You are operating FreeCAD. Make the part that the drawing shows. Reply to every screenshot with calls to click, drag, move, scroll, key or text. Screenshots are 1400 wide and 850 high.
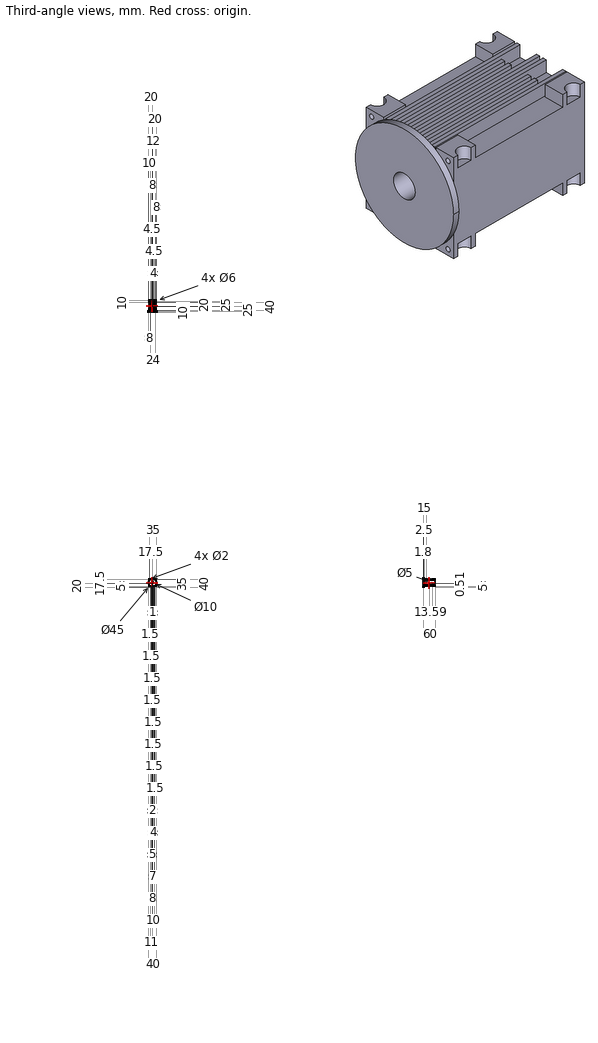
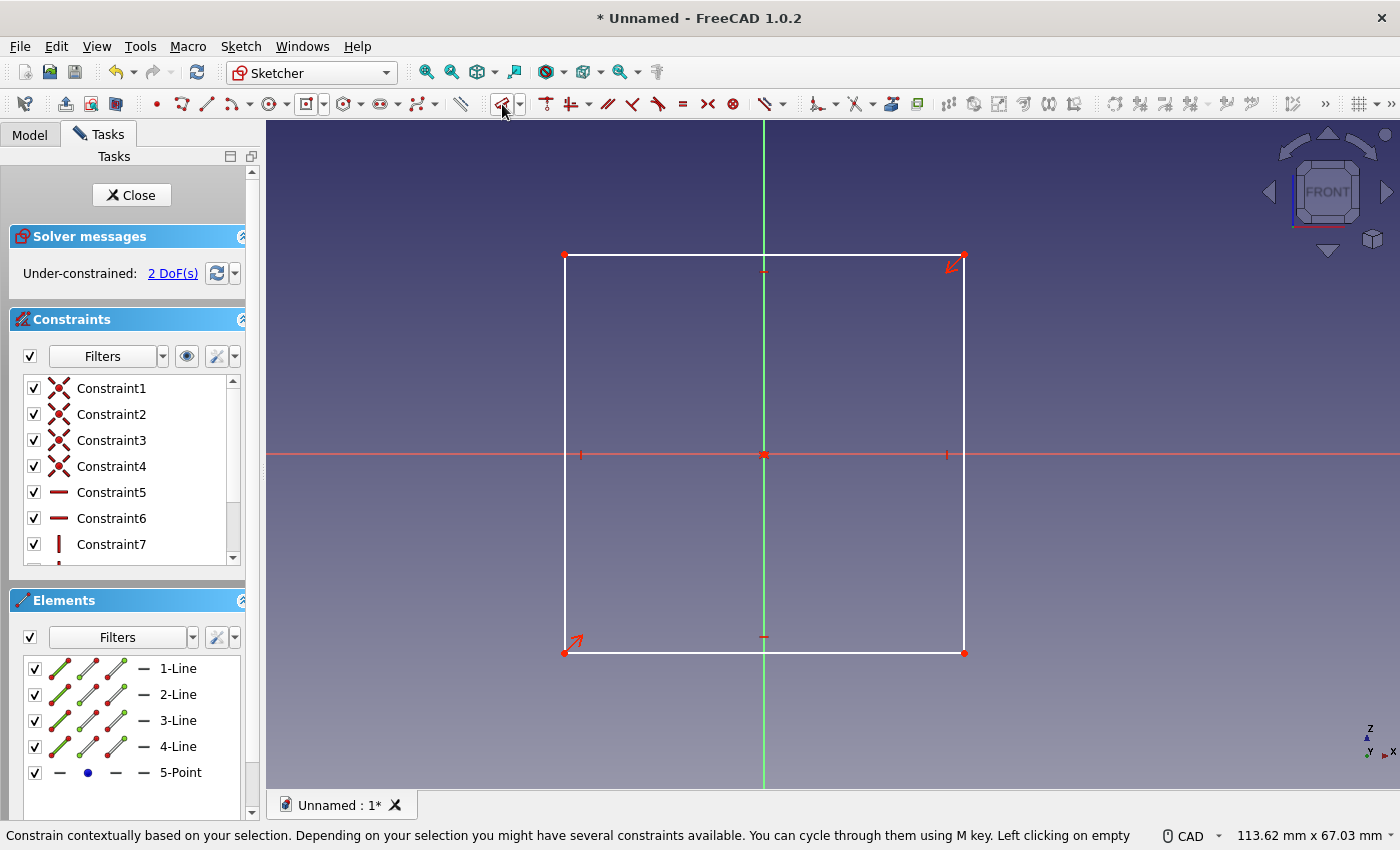
click(684, 653)
click(672, 687)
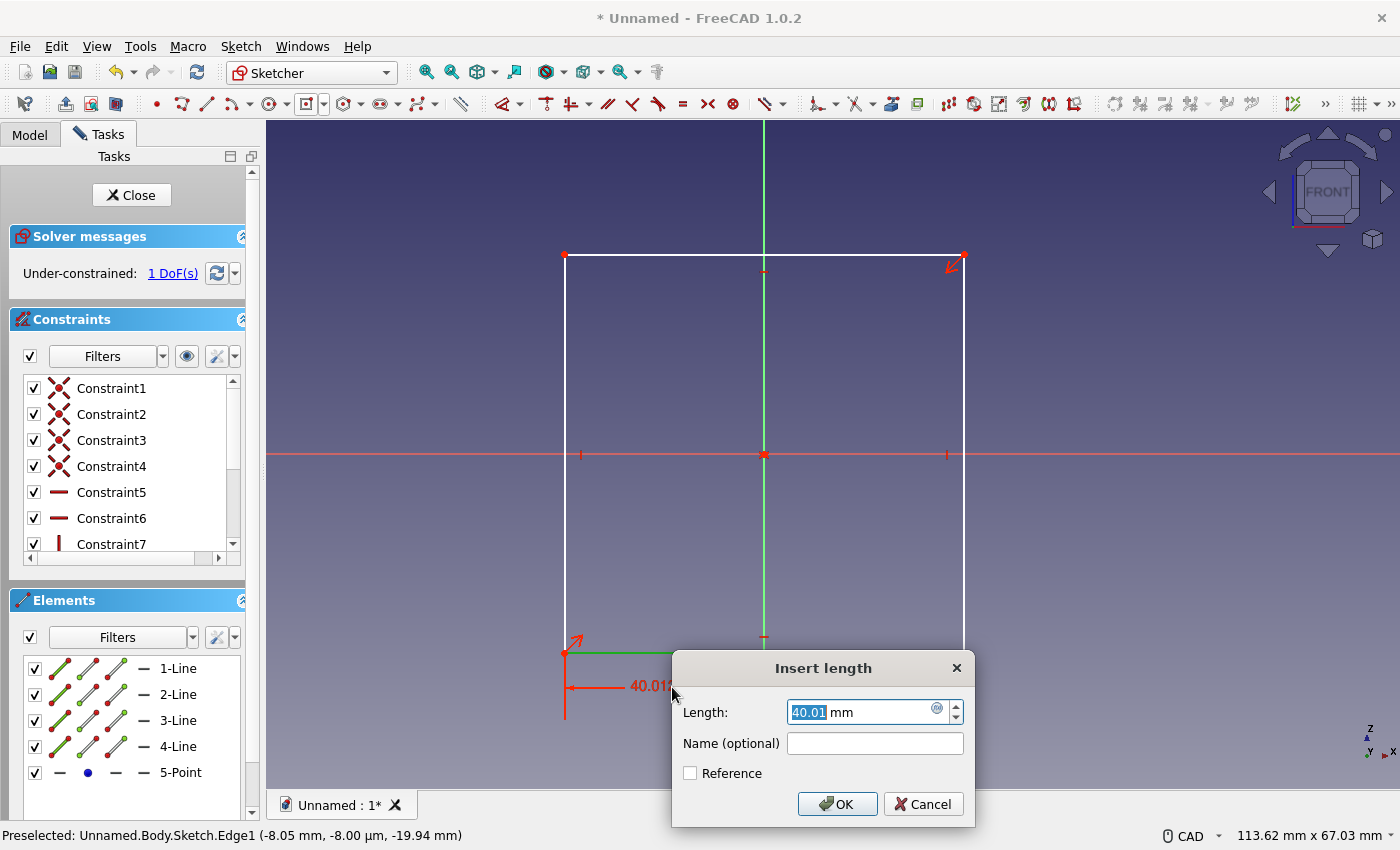
text(40)
key(Return)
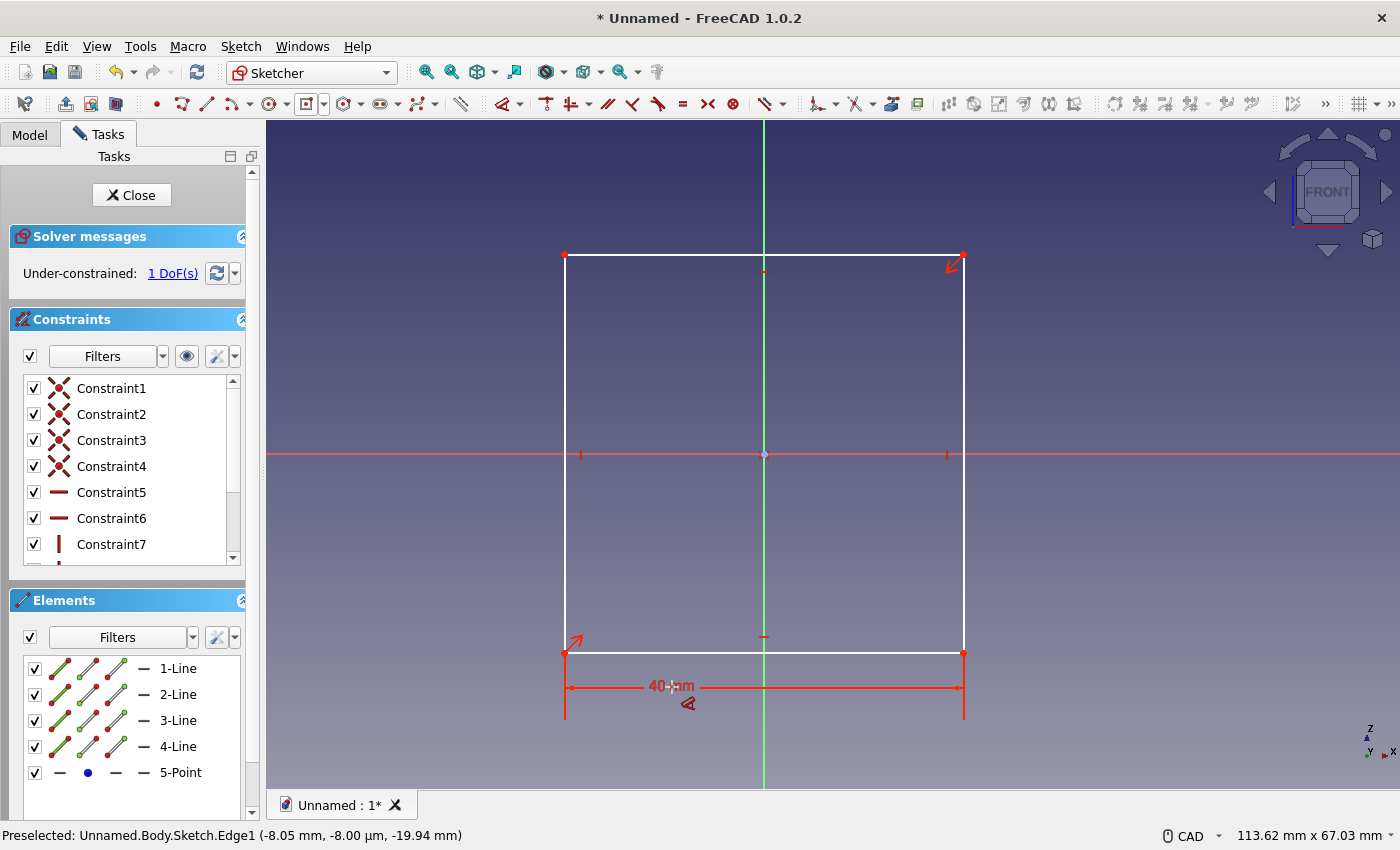
click(964, 534)
click(998, 362)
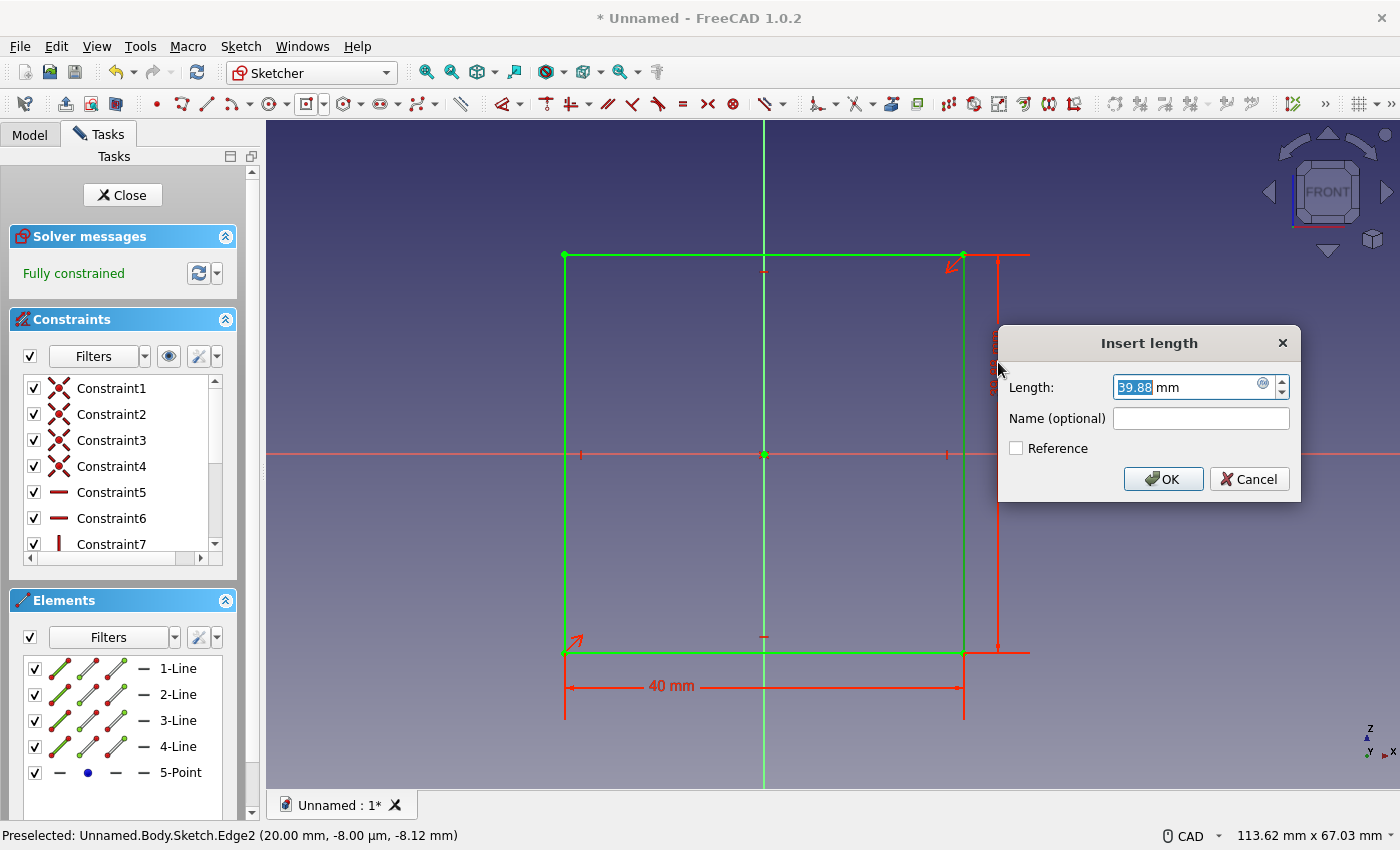
text(40)
key(Return)
key(Escape)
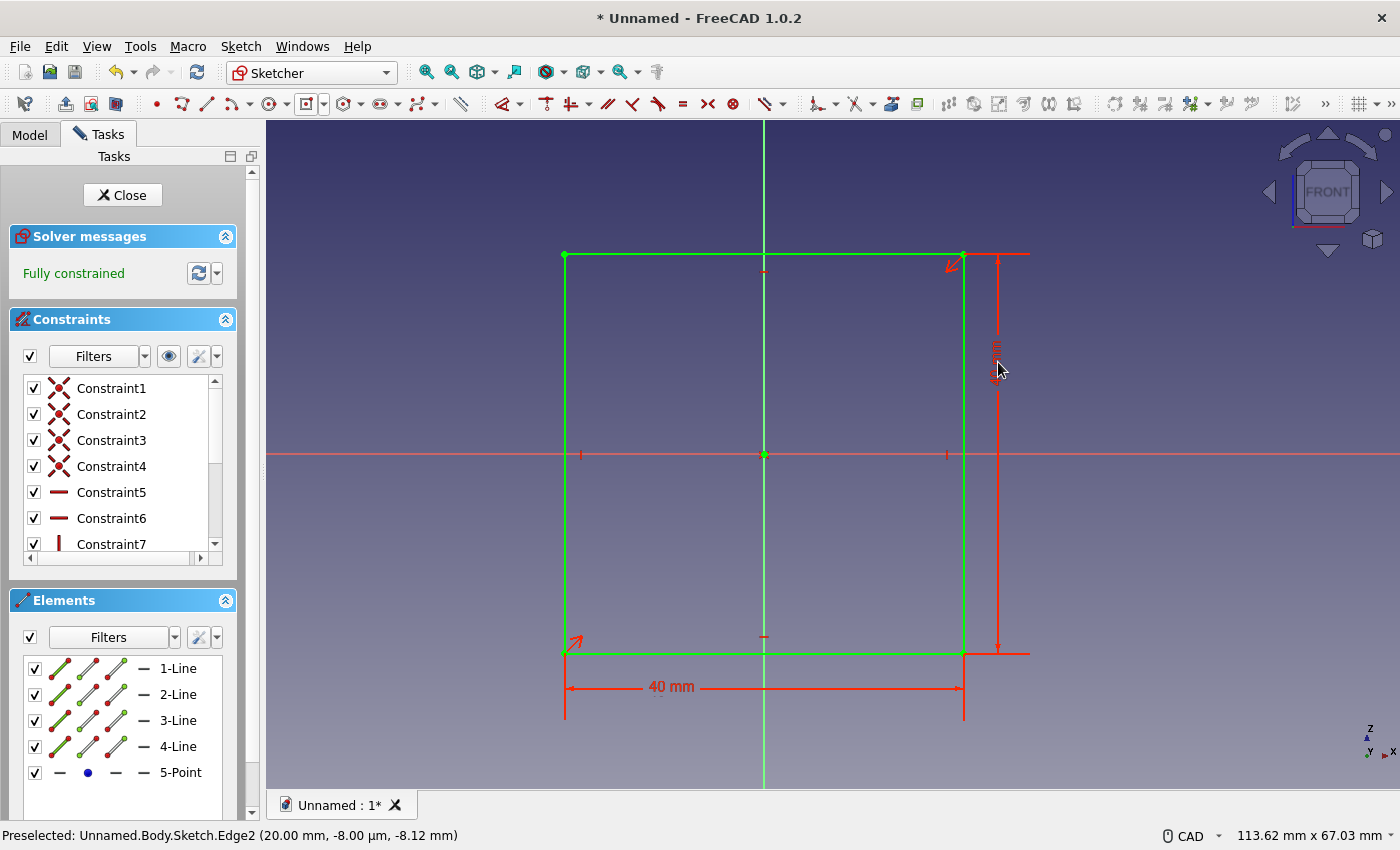
click(123, 195)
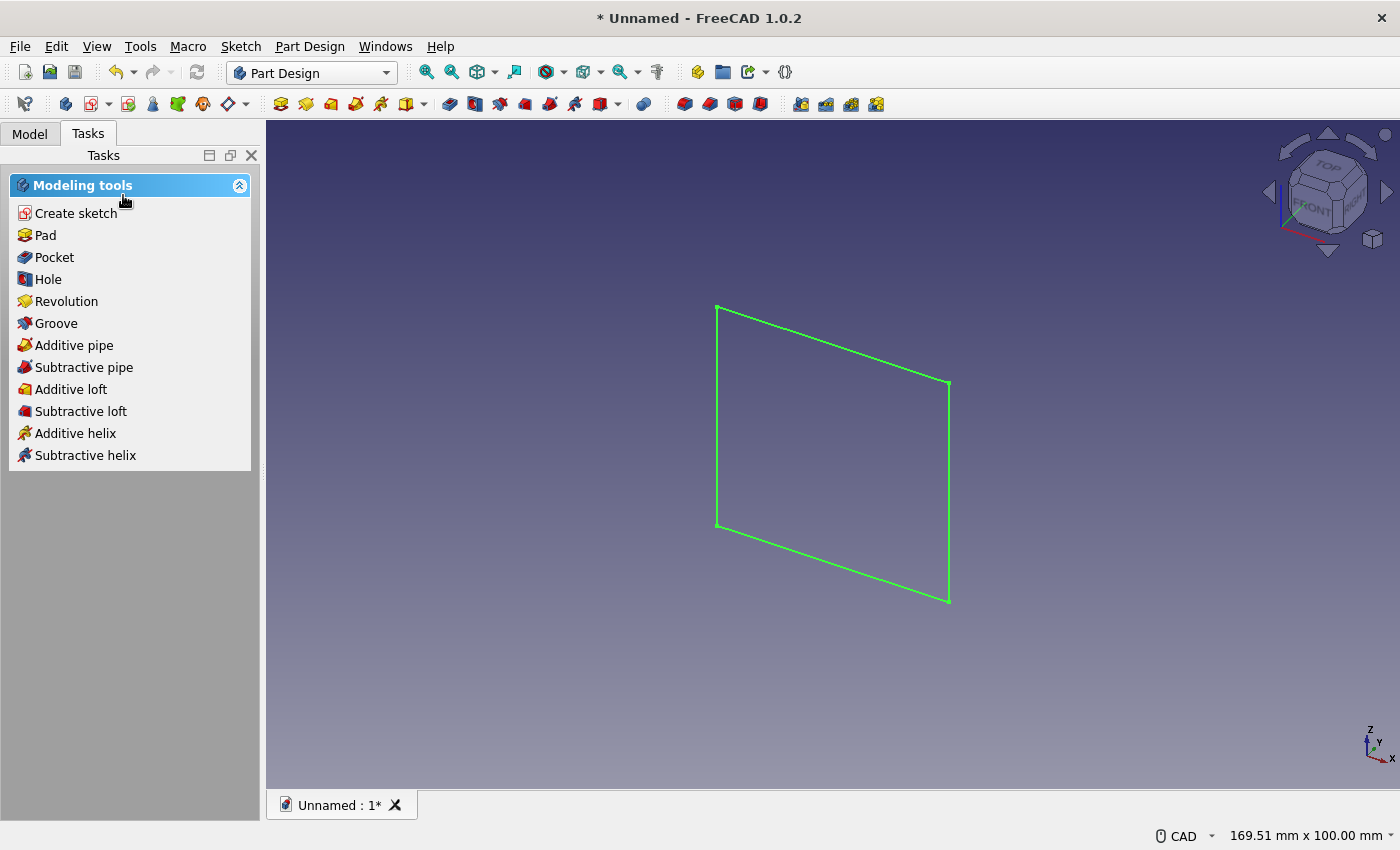
click(281, 104)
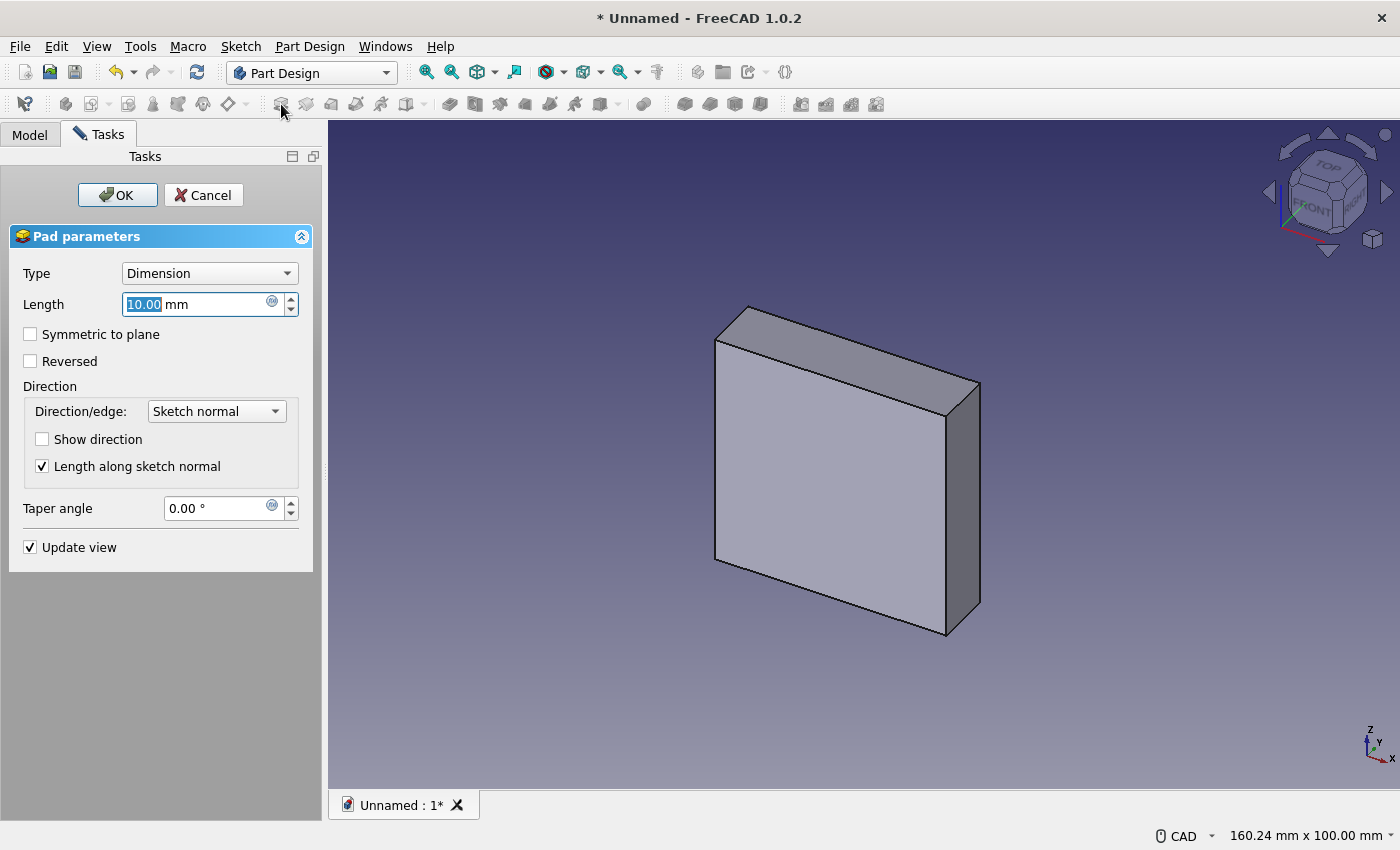
text(60)
key(Tab)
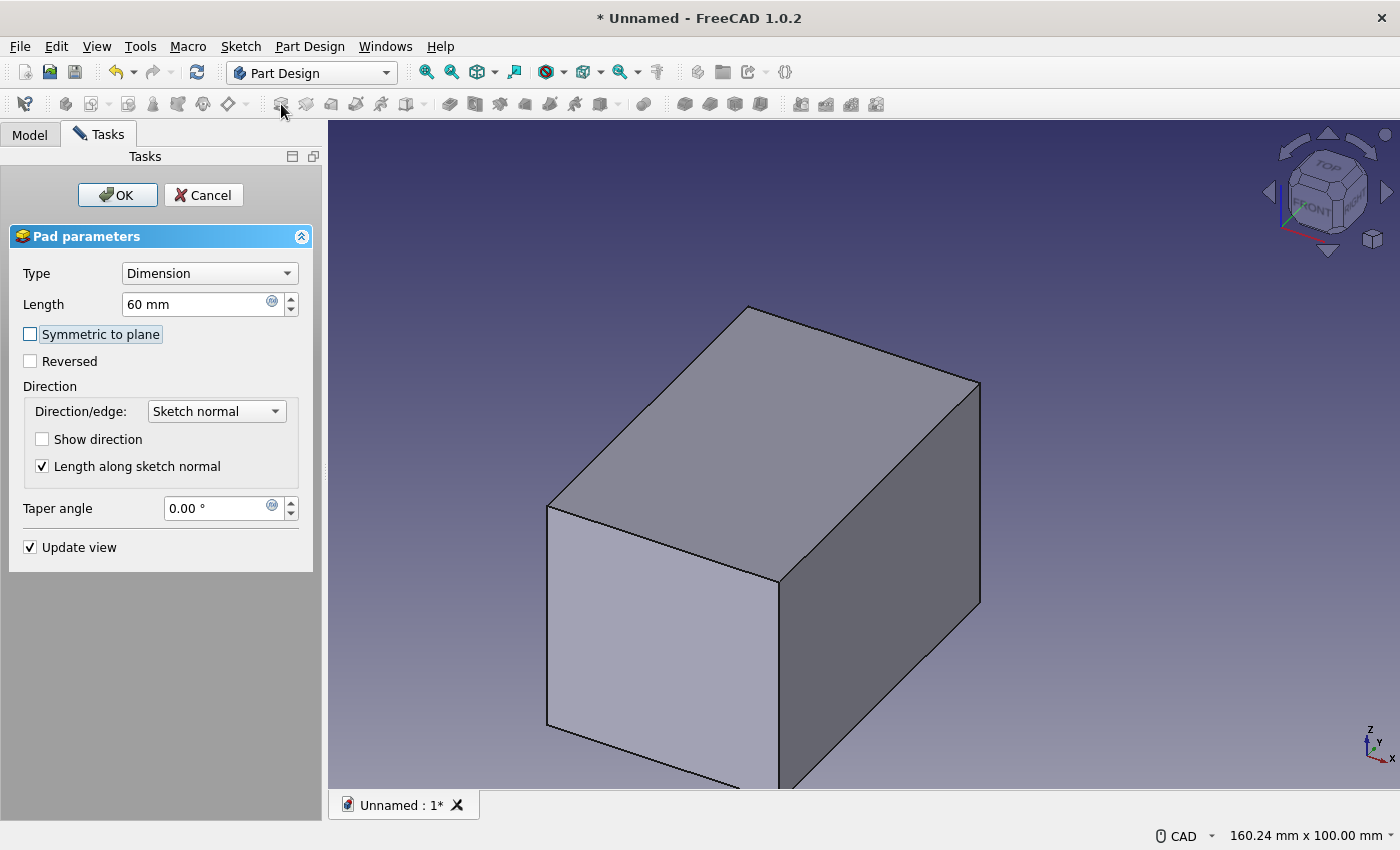
click(31, 334)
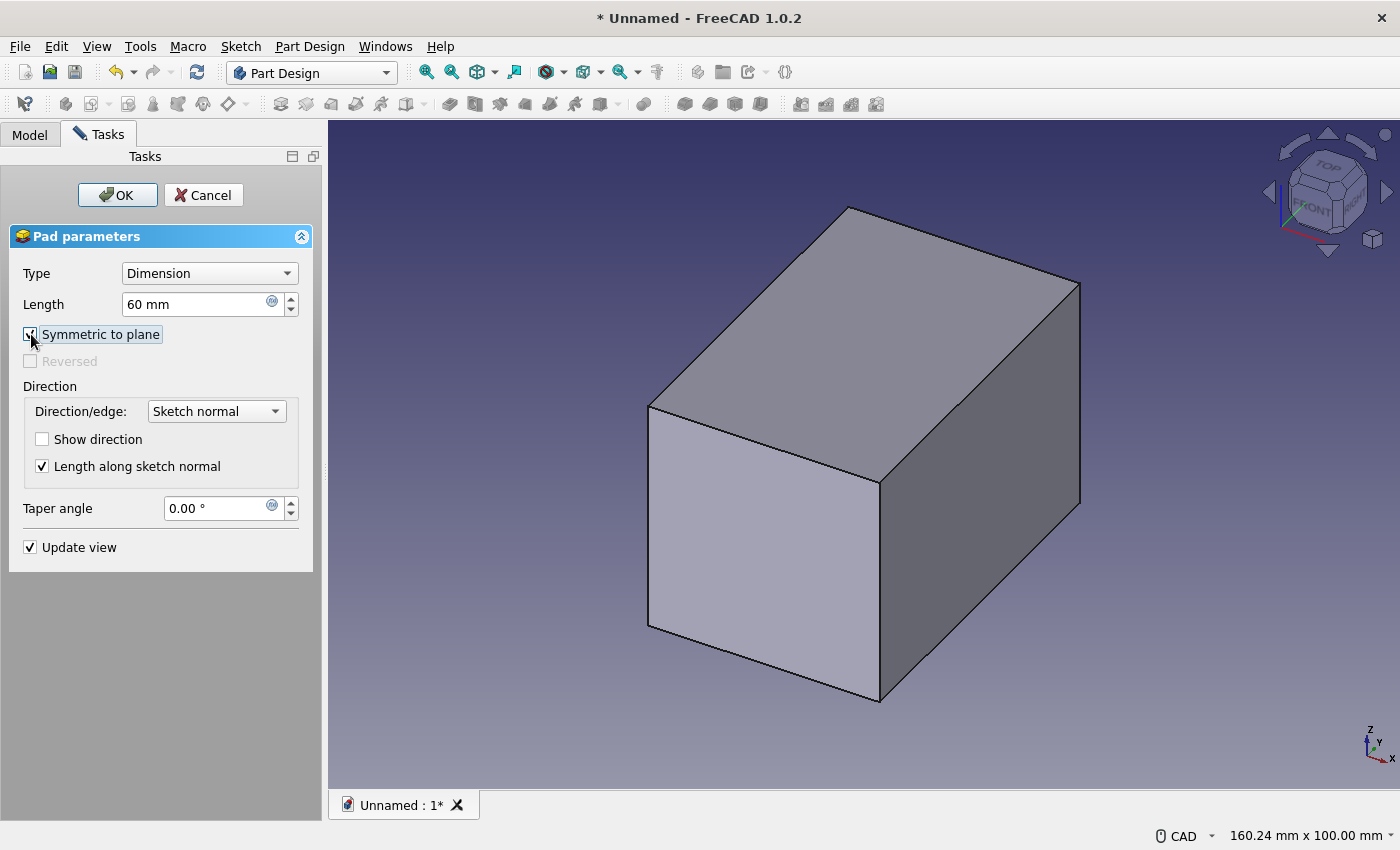
click(118, 195)